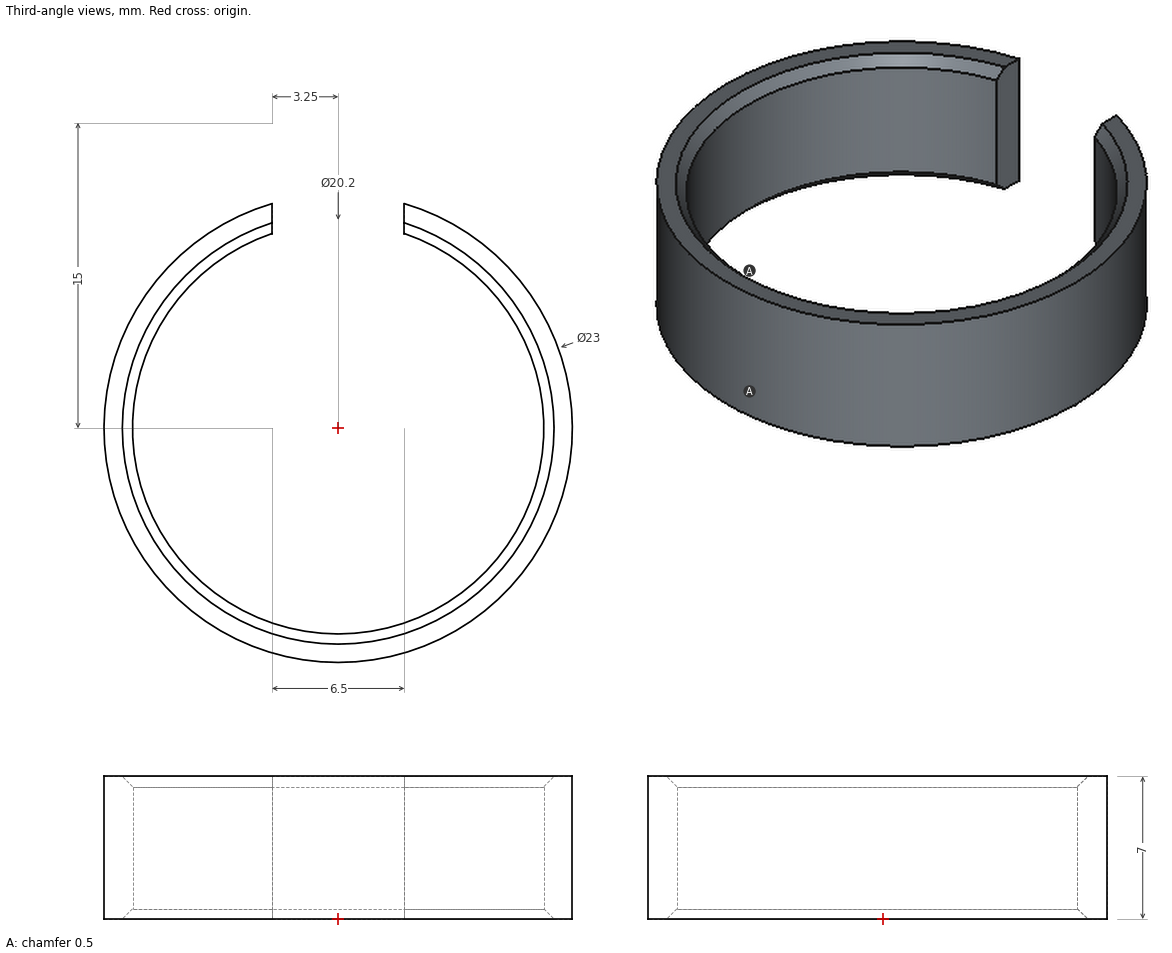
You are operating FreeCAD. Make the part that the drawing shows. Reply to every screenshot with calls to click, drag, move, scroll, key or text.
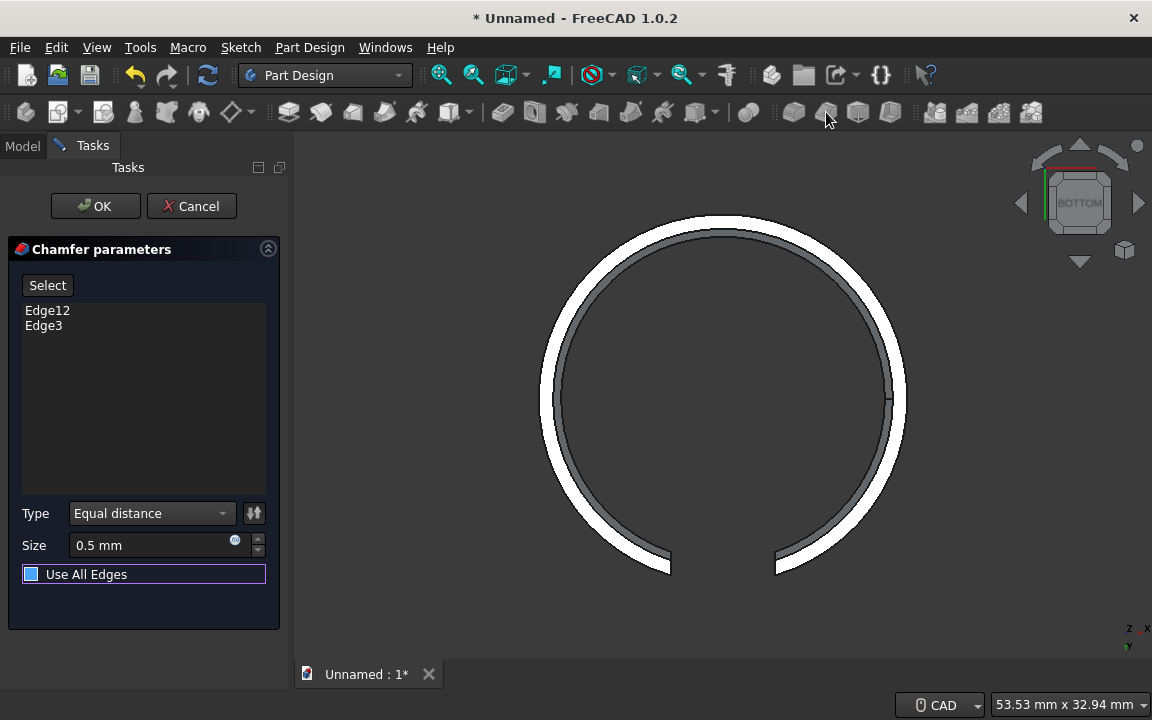
click(96, 206)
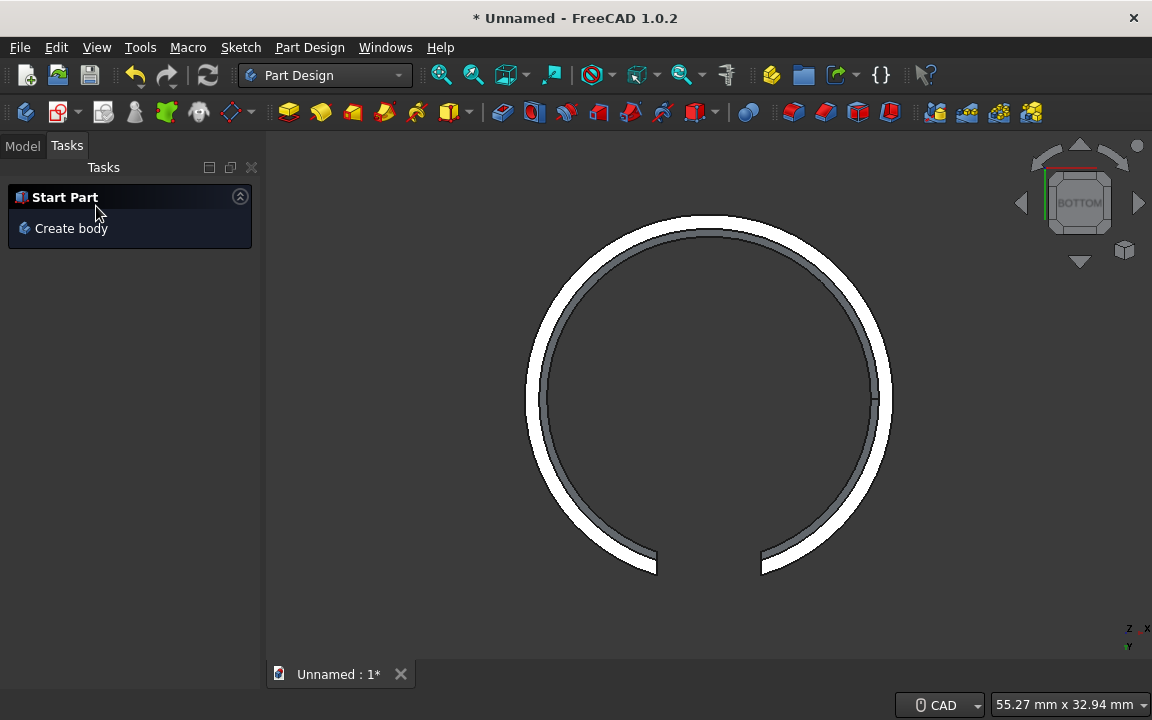
key(0)